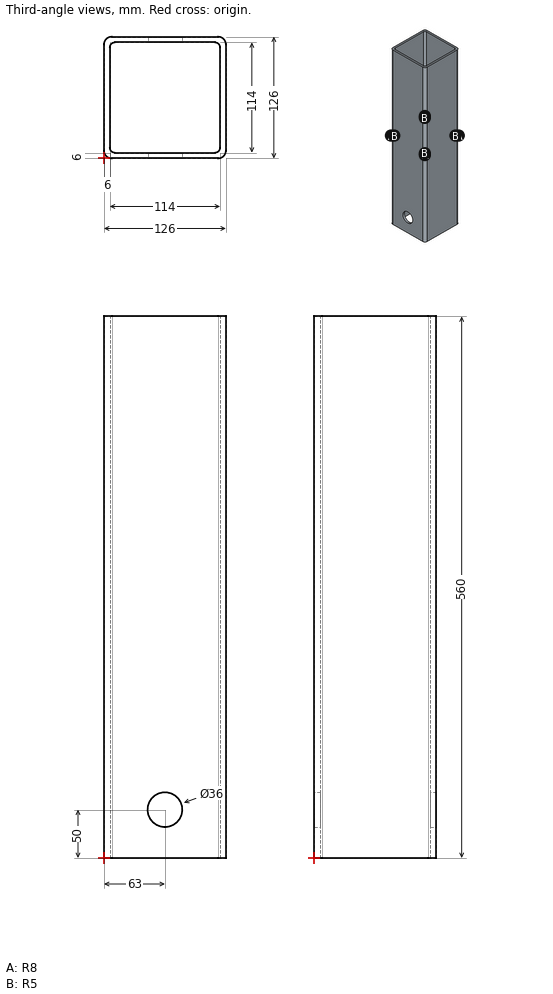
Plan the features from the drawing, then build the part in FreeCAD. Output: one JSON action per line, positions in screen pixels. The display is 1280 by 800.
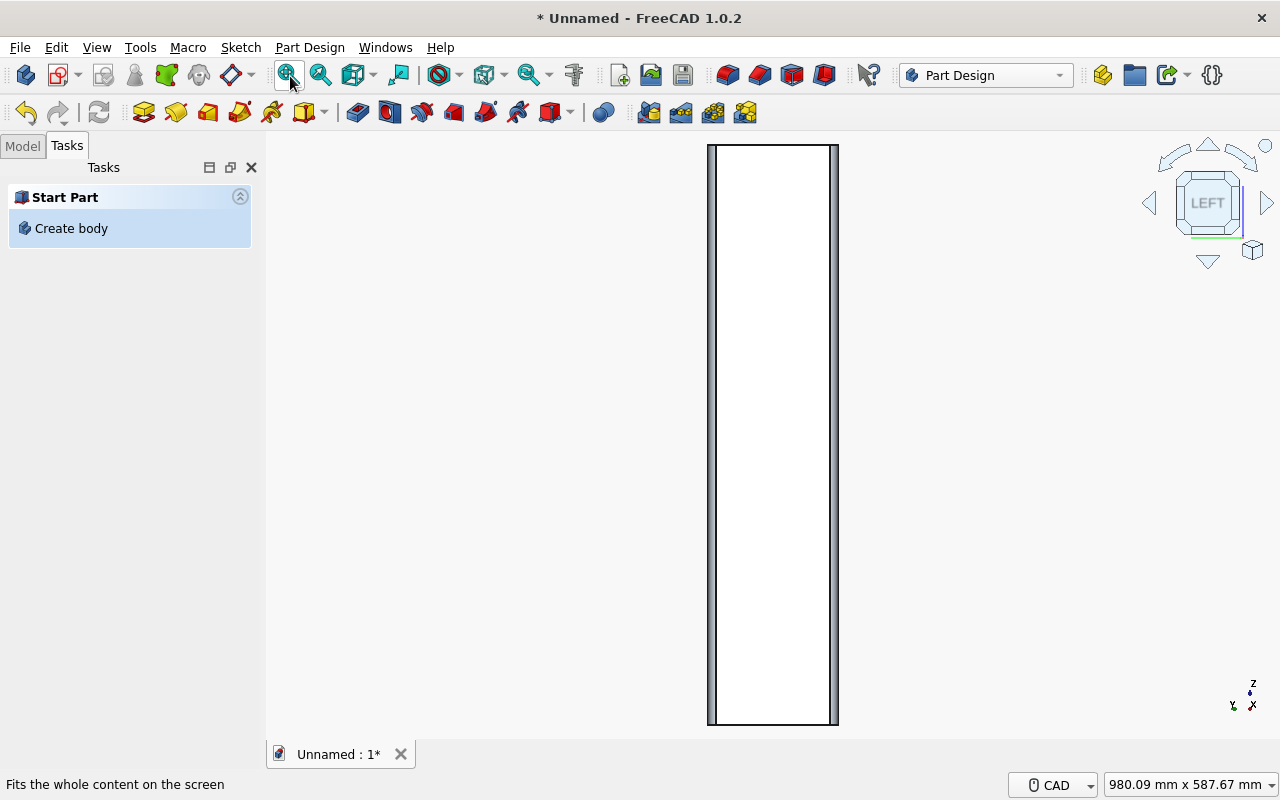
{"action": "key", "text": "v 3"}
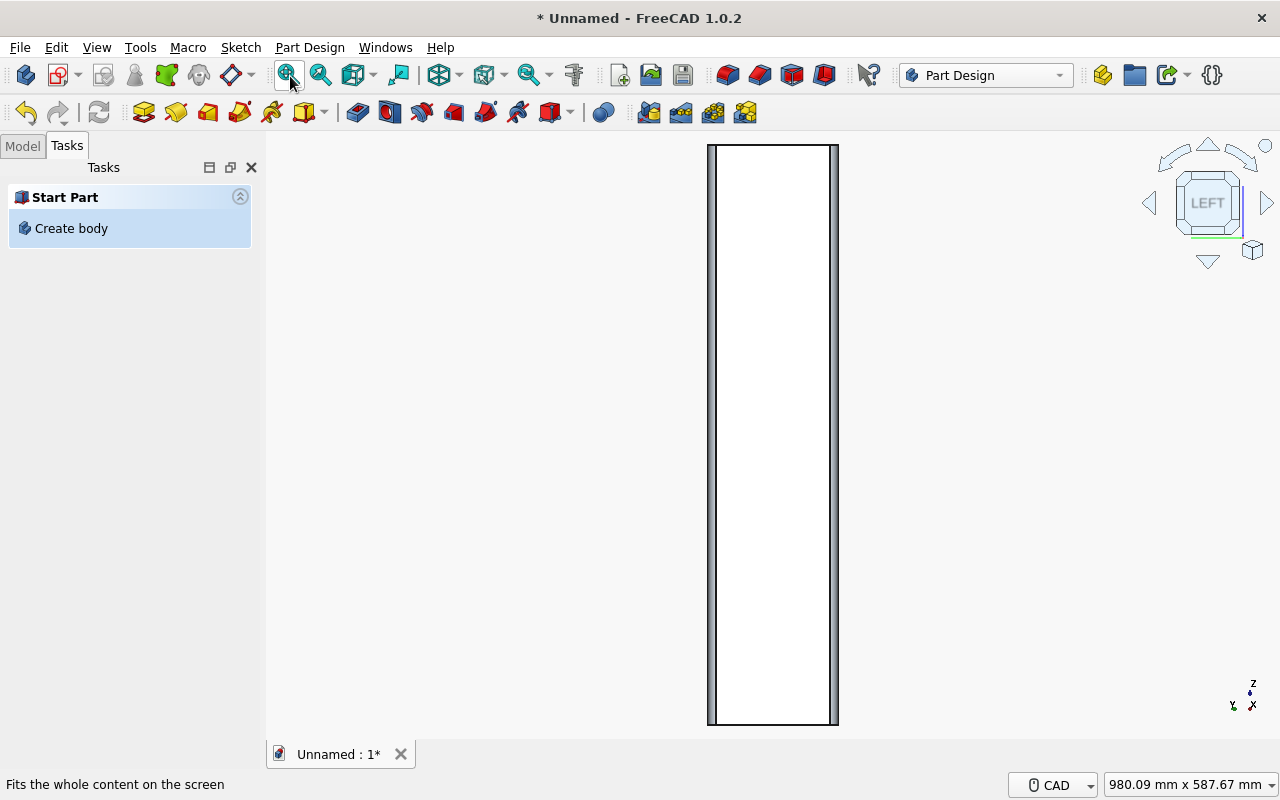
{"action": "key", "text": "0"}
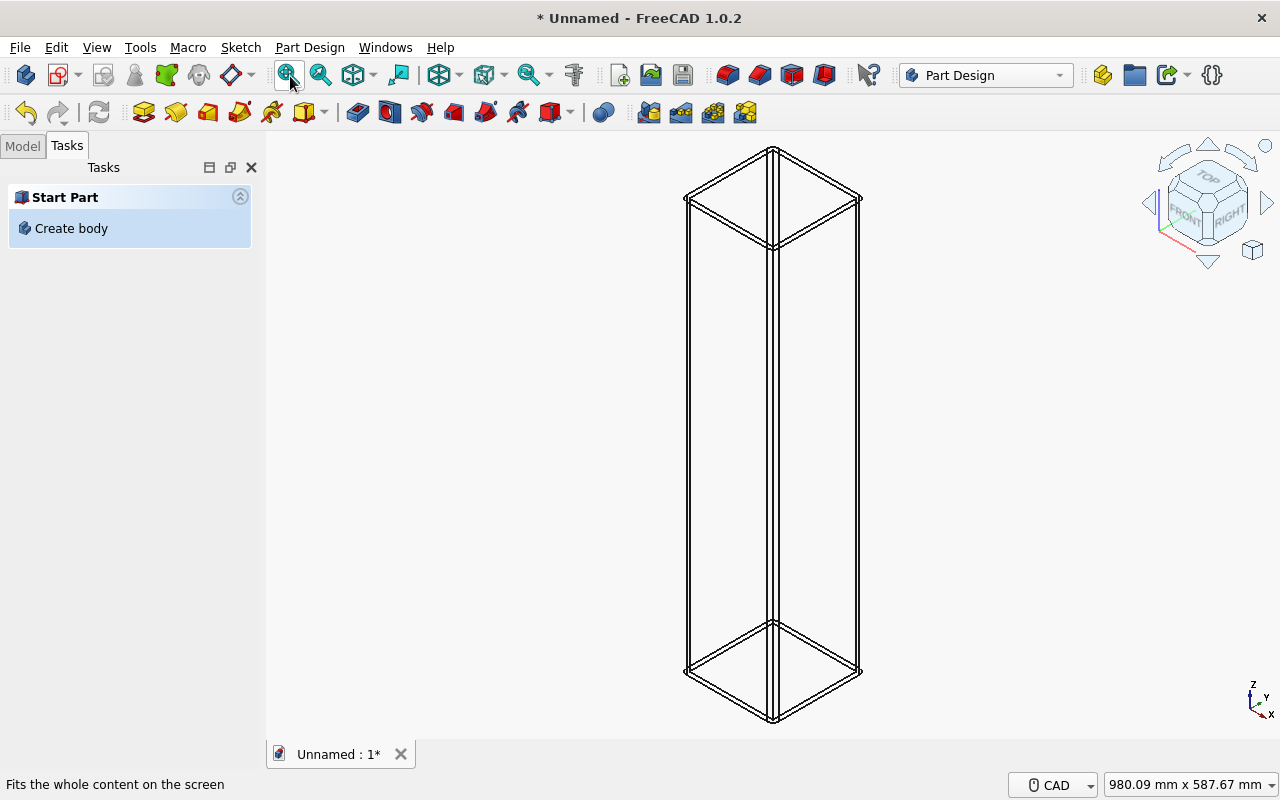
{"action": "left_click", "coordinate": [773, 206]}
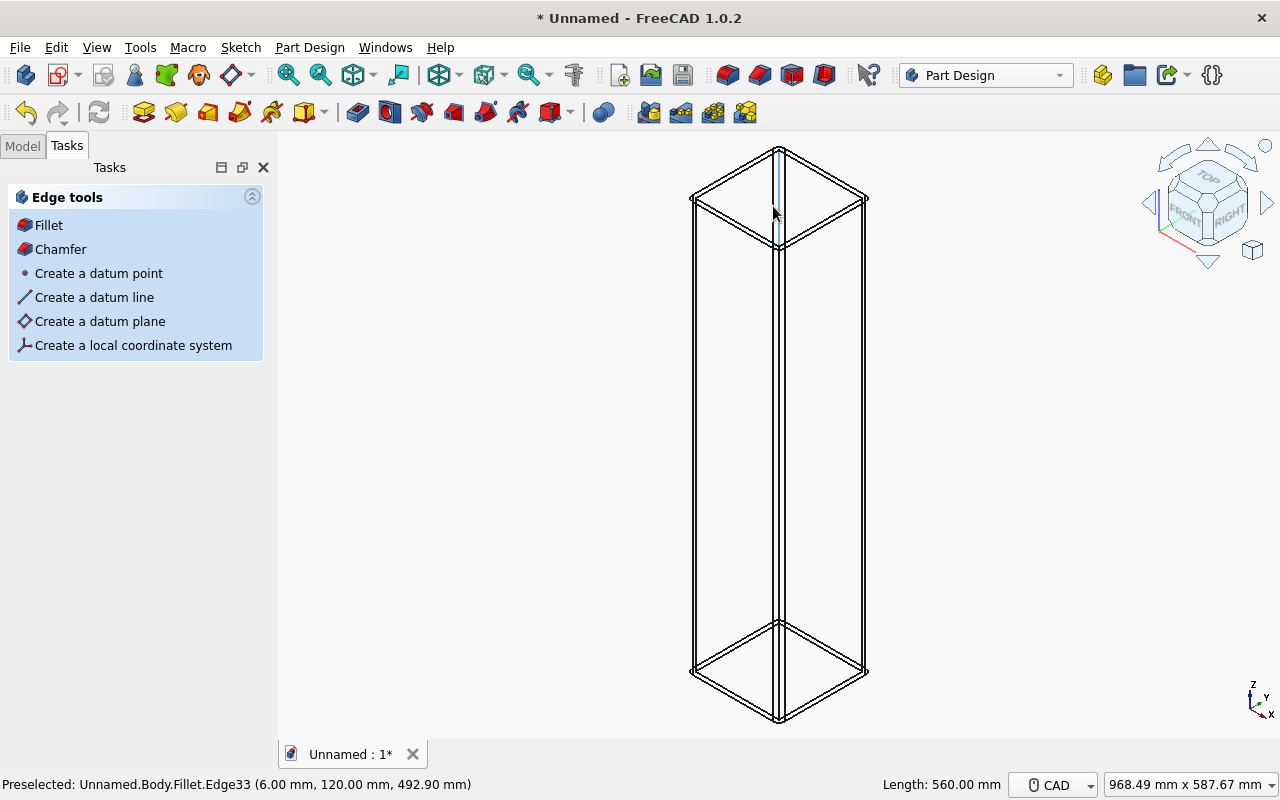
{"action": "scroll", "coordinate": [696, 434], "scroll_direction": "up", "scroll_amount": 6}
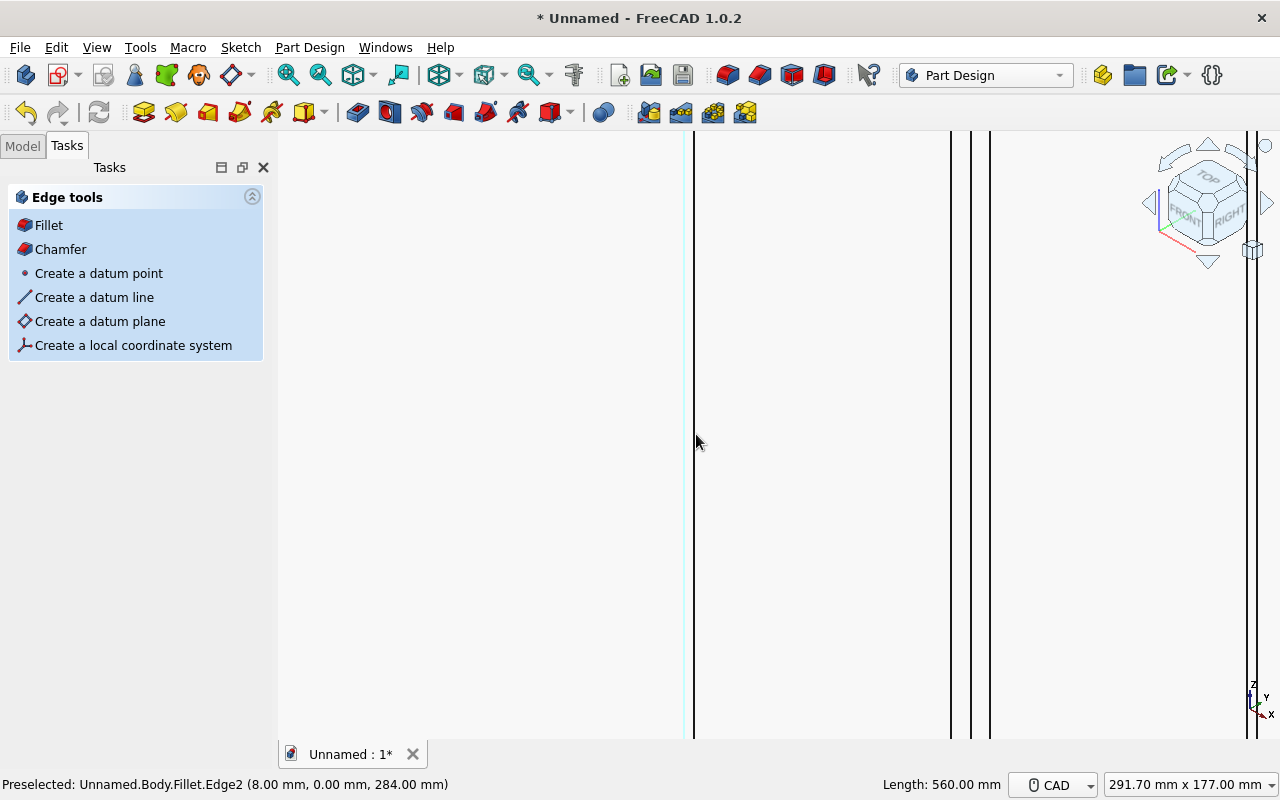
{"action": "left_click", "coordinate": [694, 435], "text": "ctrl"}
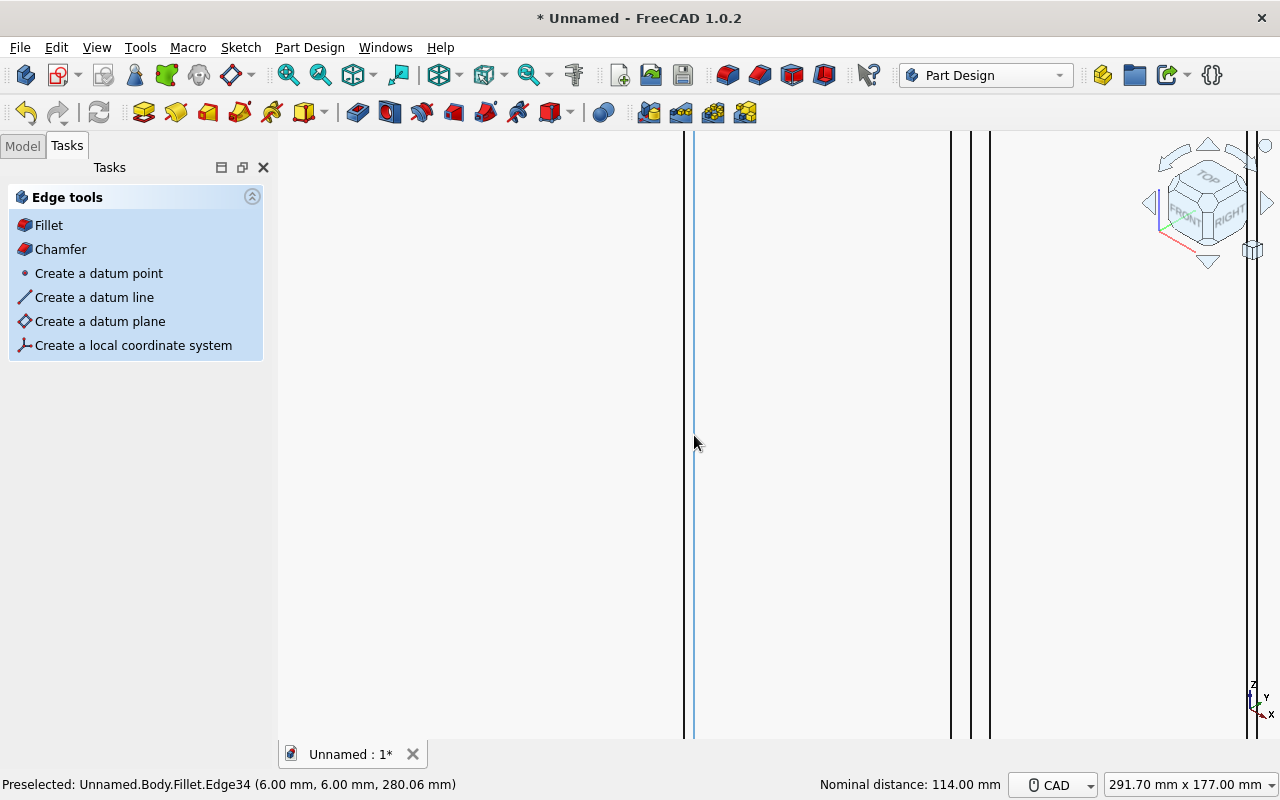
{"action": "left_click", "coordinate": [971, 595], "text": "ctrl"}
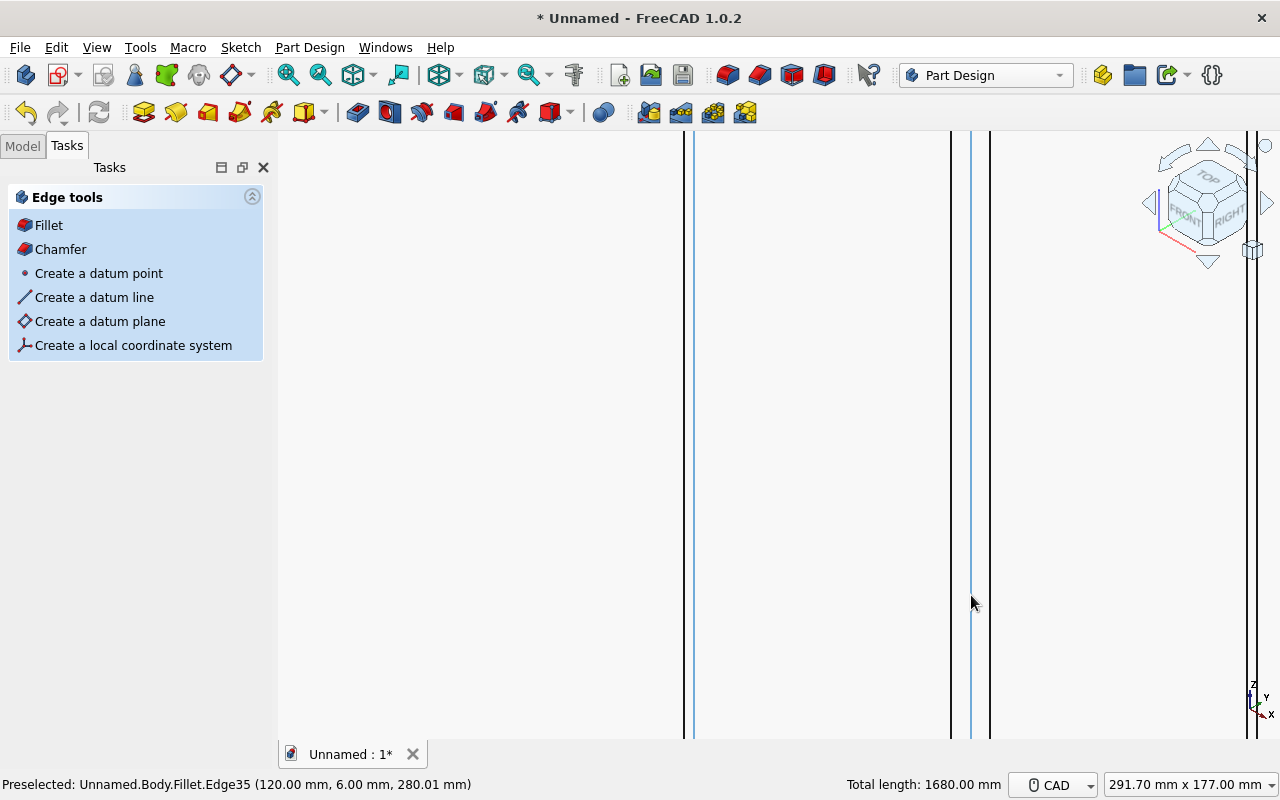
{"action": "left_click", "coordinate": [290, 76]}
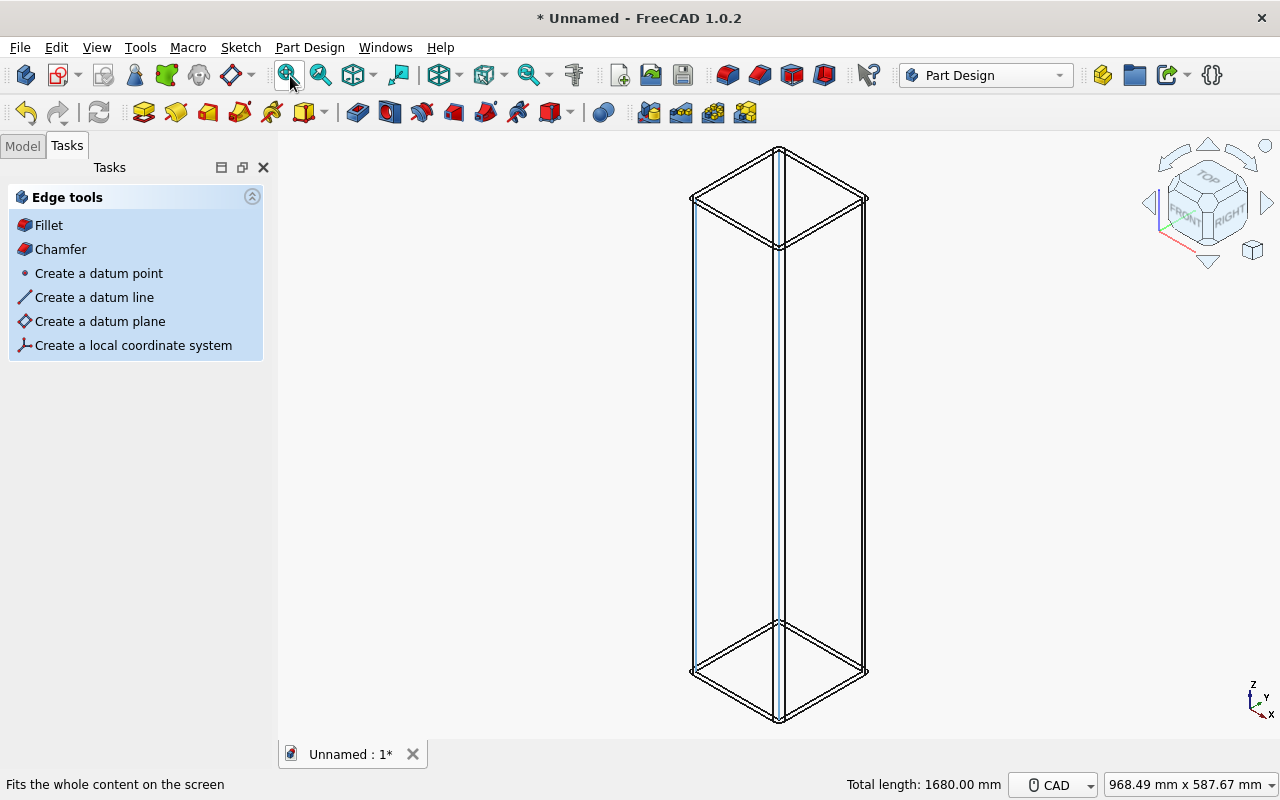
{"action": "key", "text": "2"}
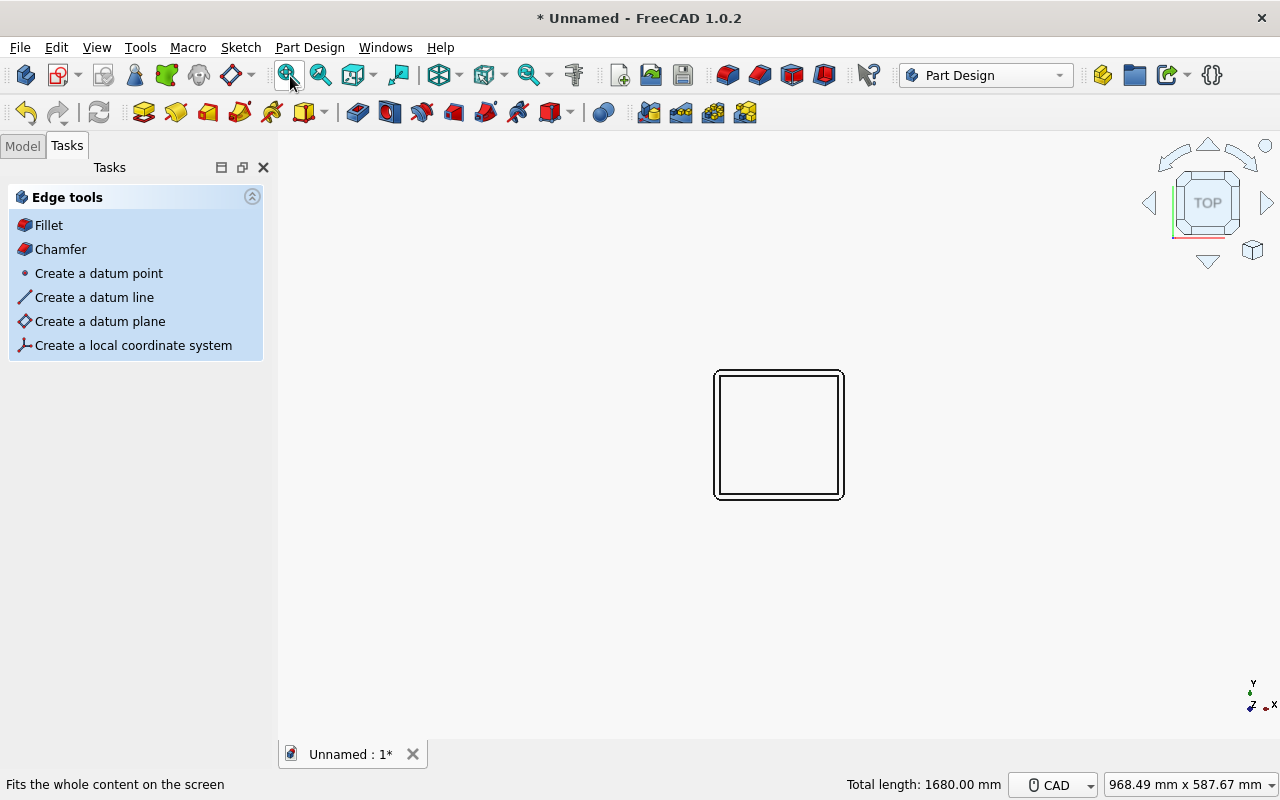
{"action": "left_click", "coordinate": [290, 76]}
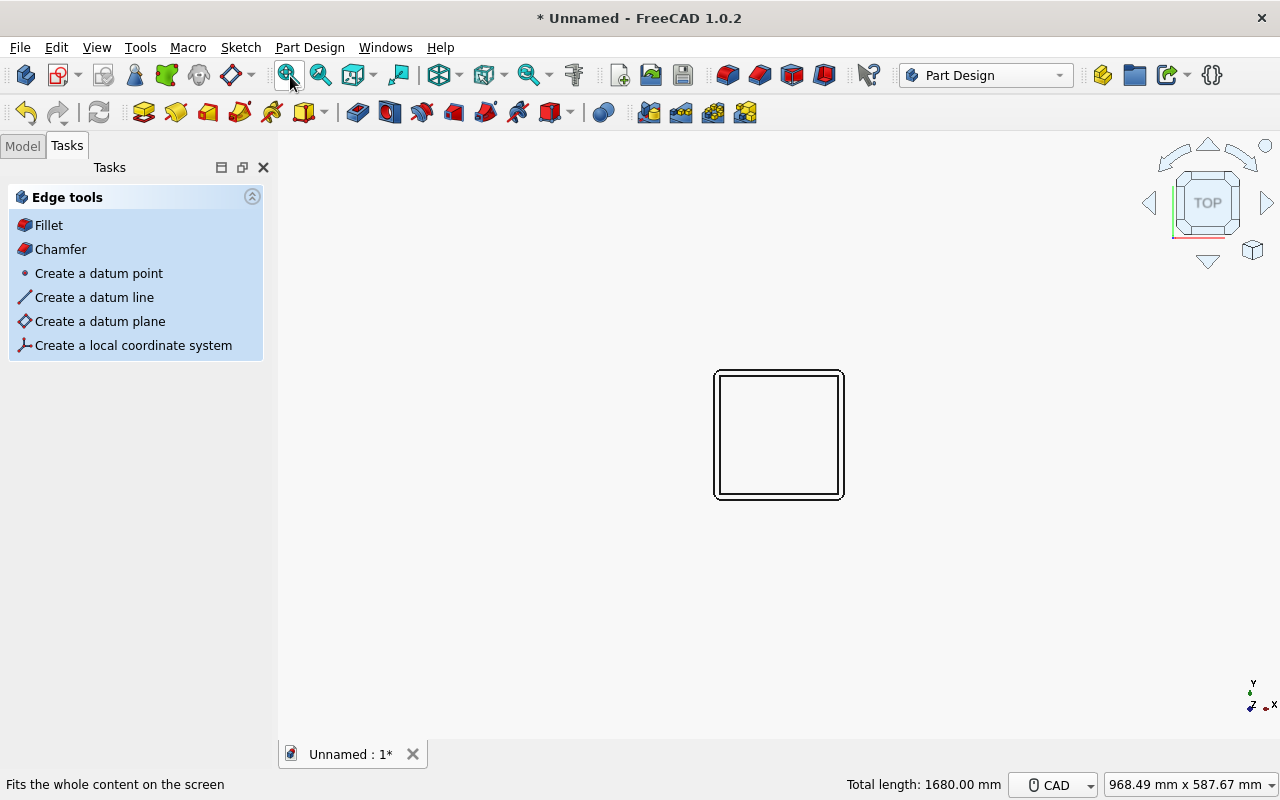
{"action": "scroll", "coordinate": [838, 375], "scroll_direction": "up", "scroll_amount": 6}